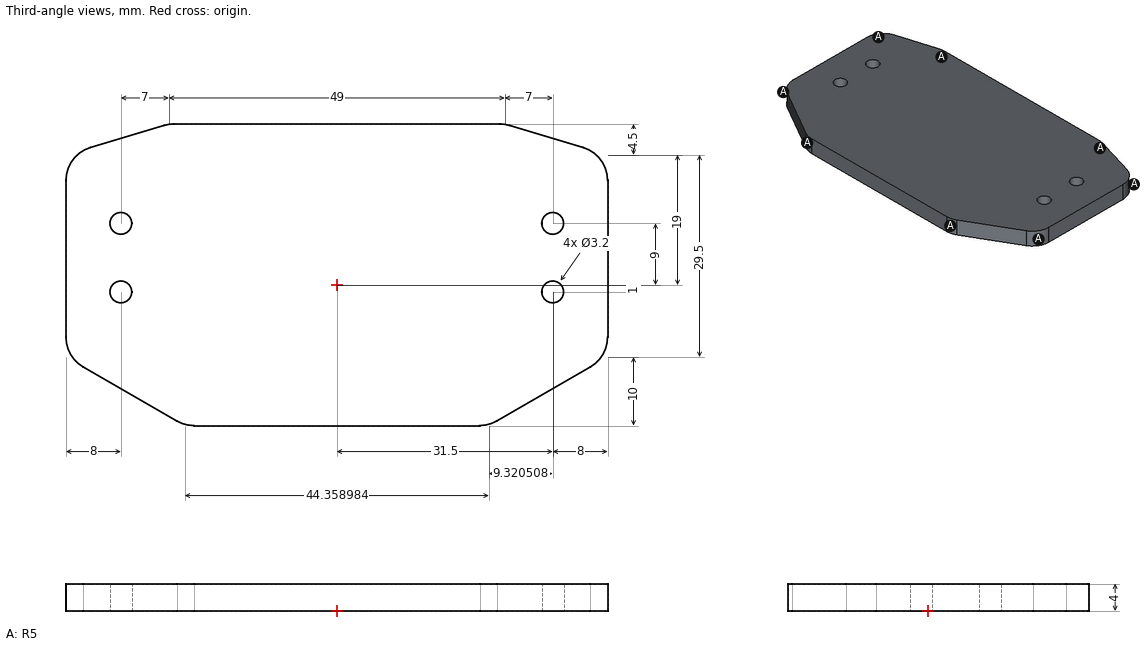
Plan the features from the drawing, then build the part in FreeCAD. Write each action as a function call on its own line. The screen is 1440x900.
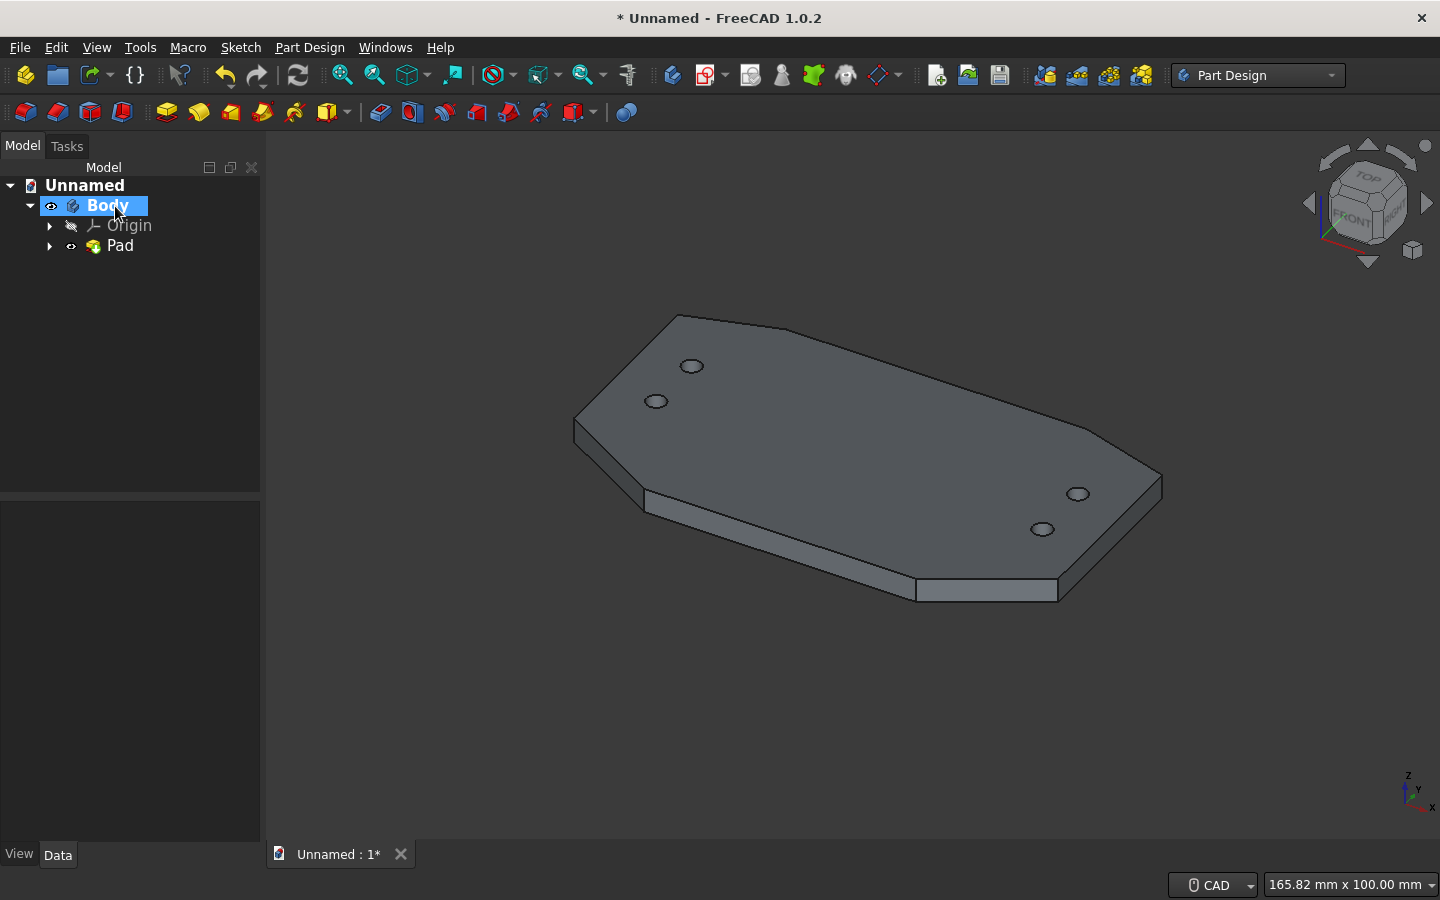
click(916, 590)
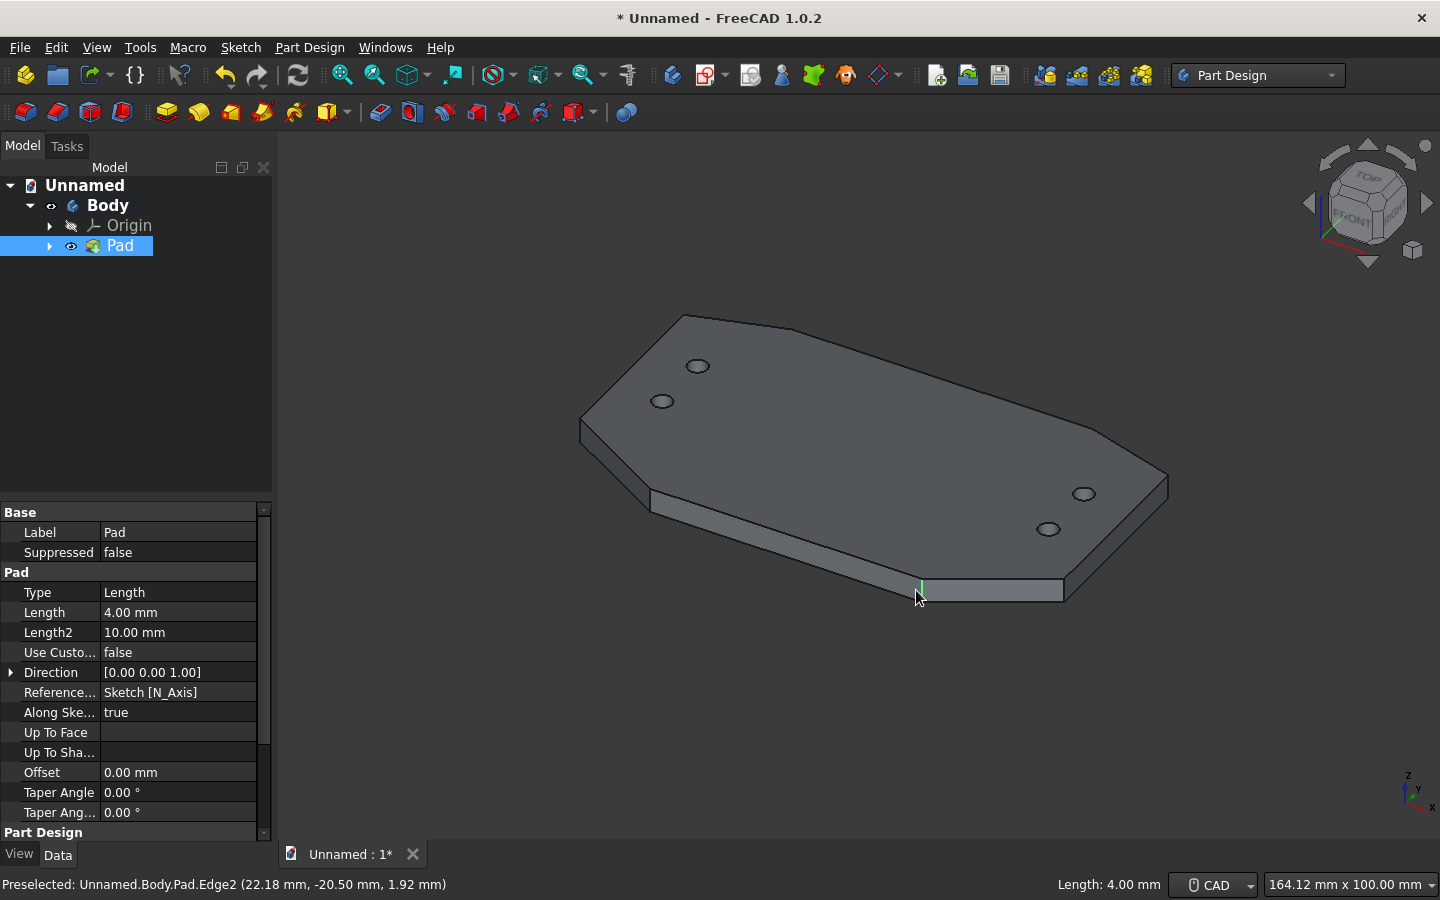
key(0)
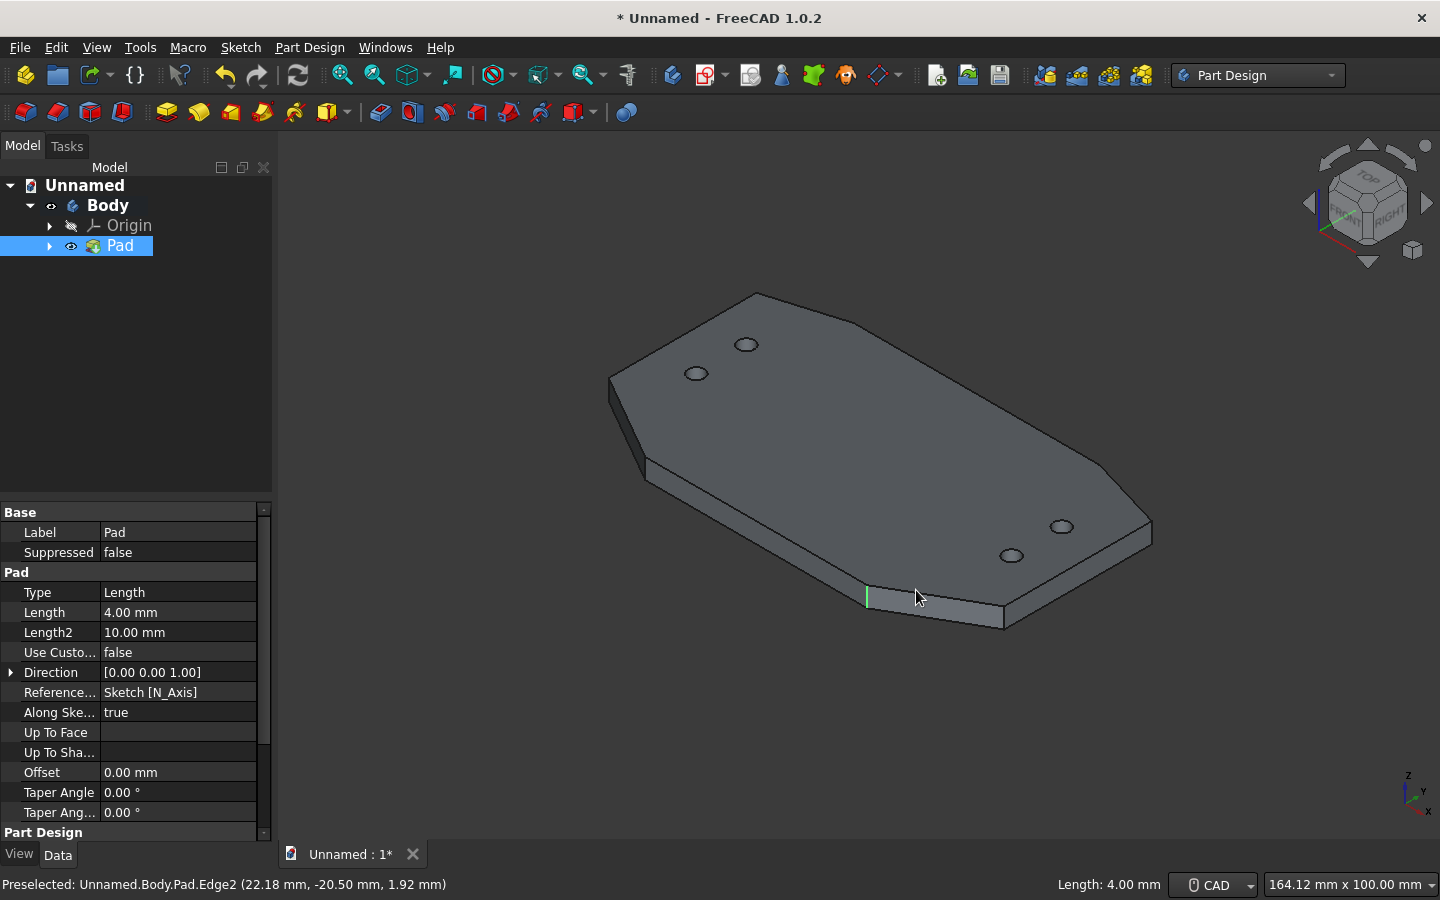
click(1004, 617, ctrl)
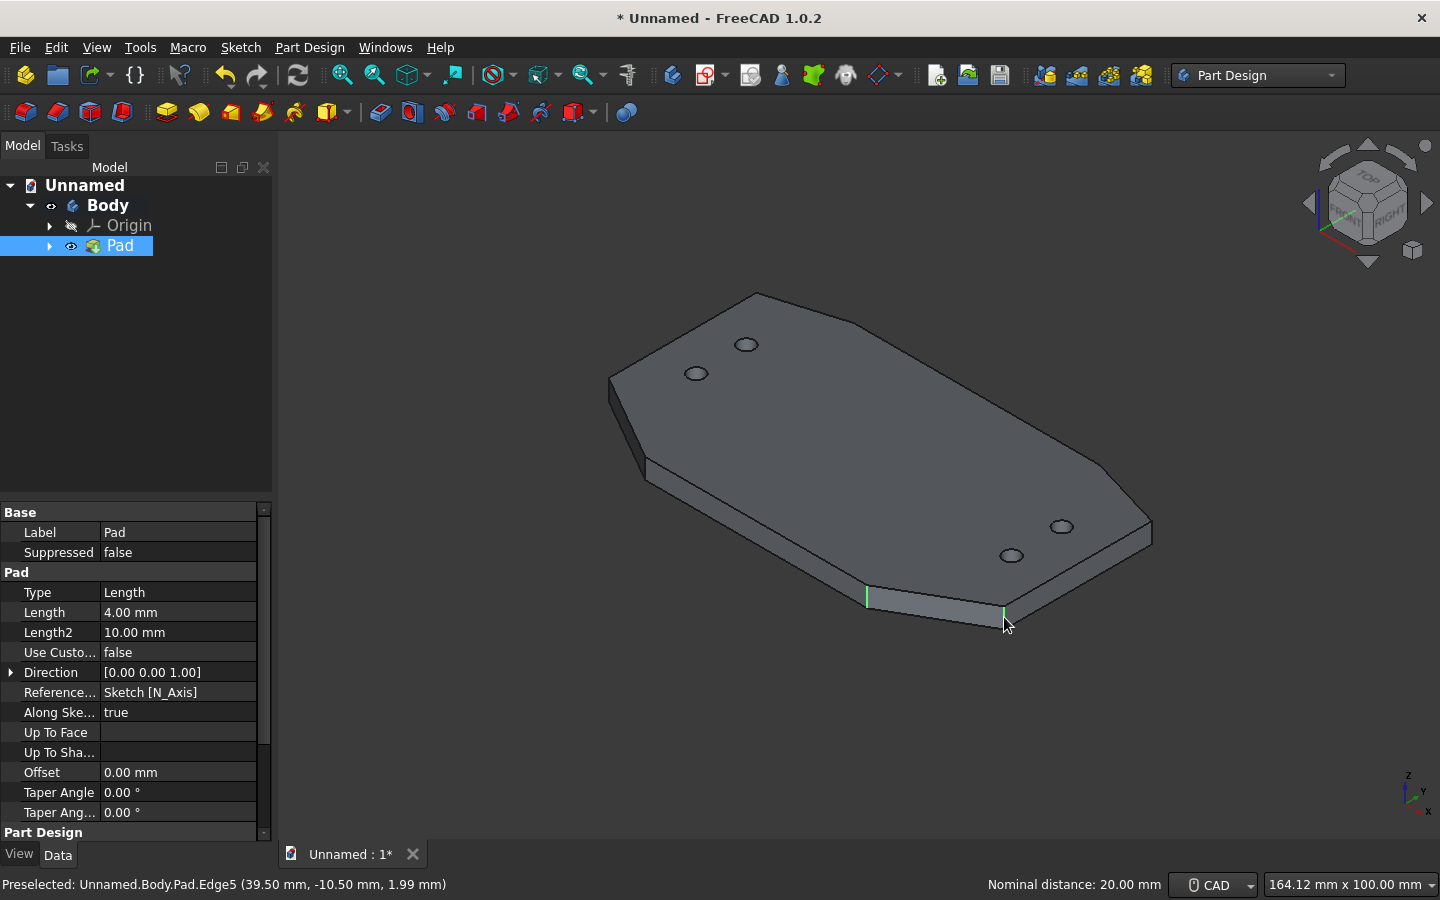
key(2)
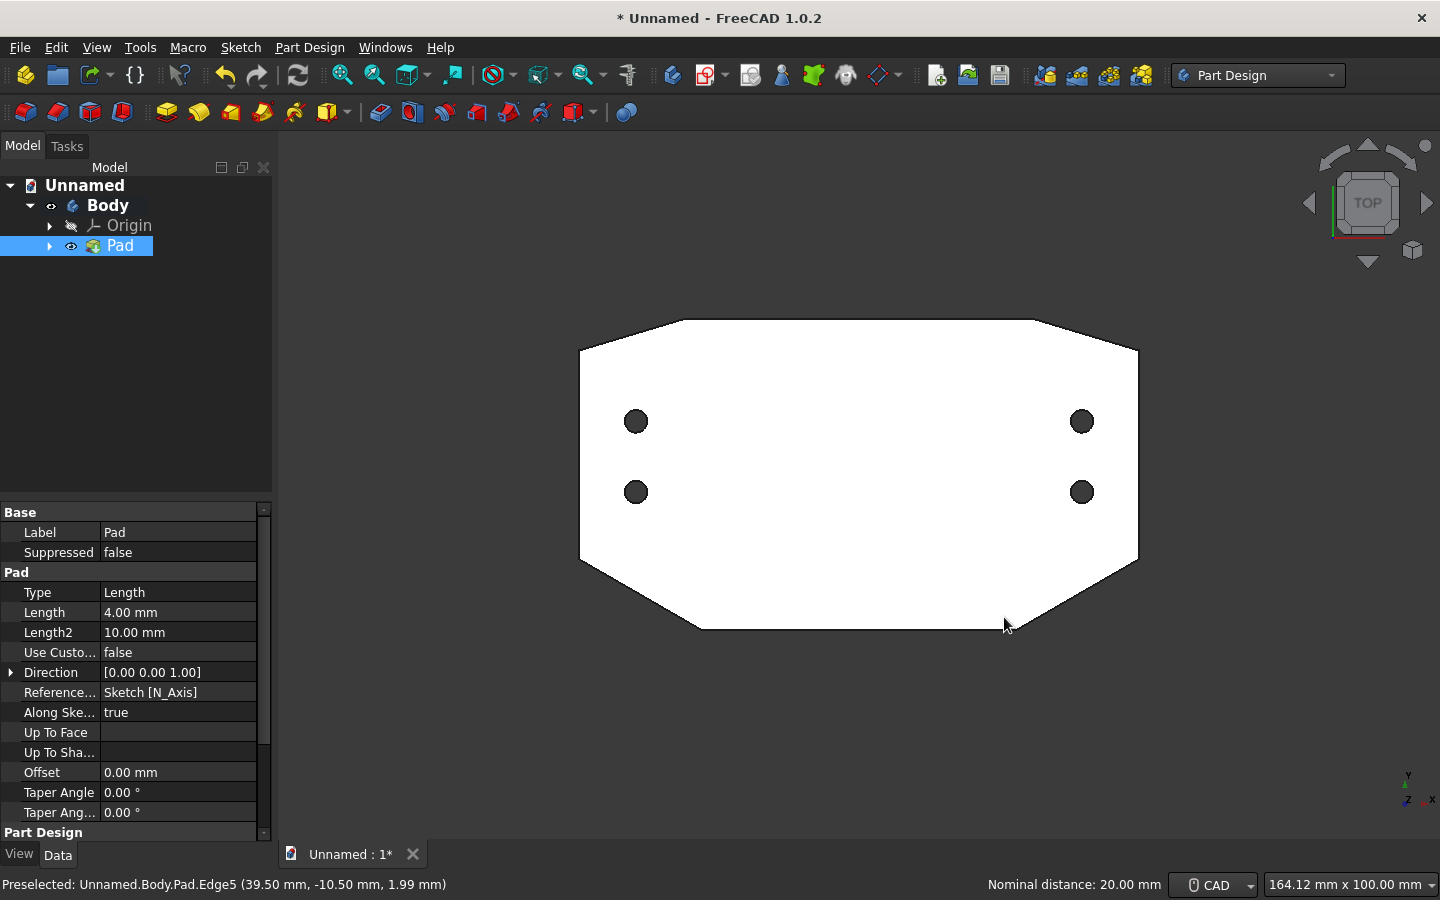
key(1)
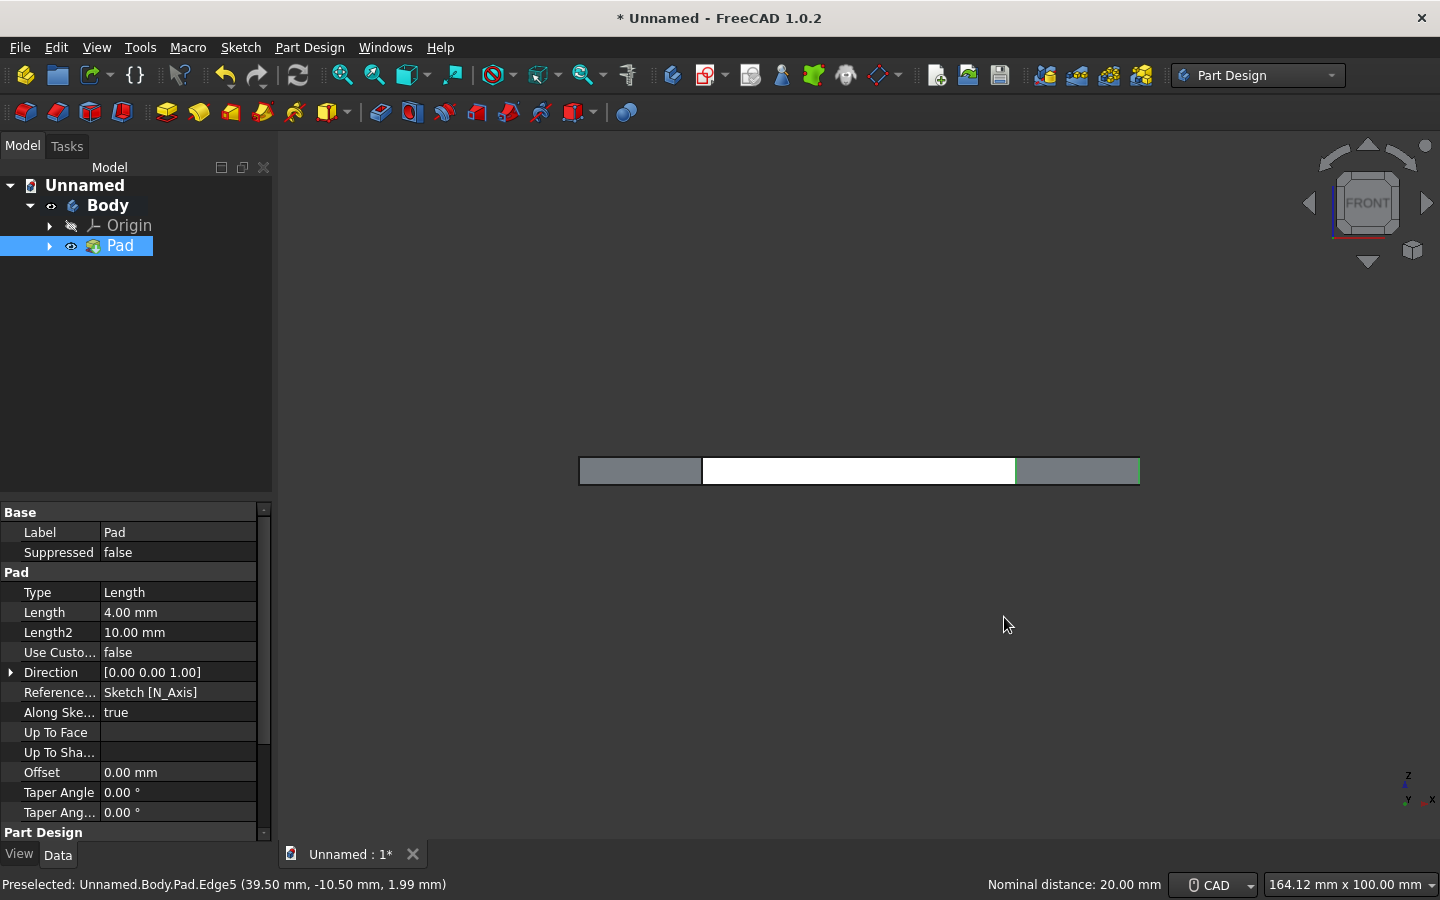
click(702, 470, ctrl)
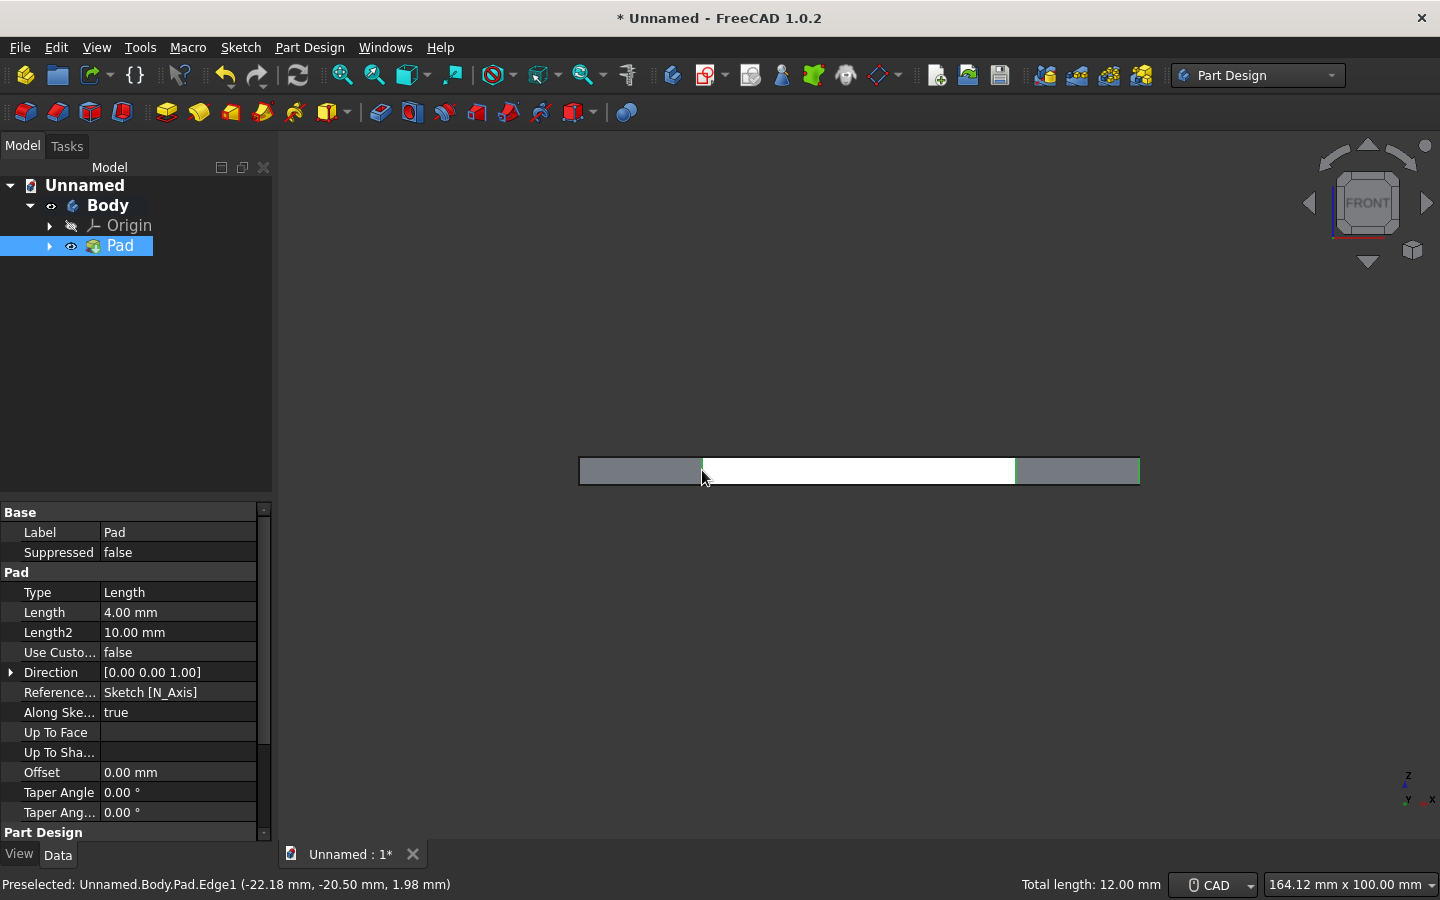
key(3)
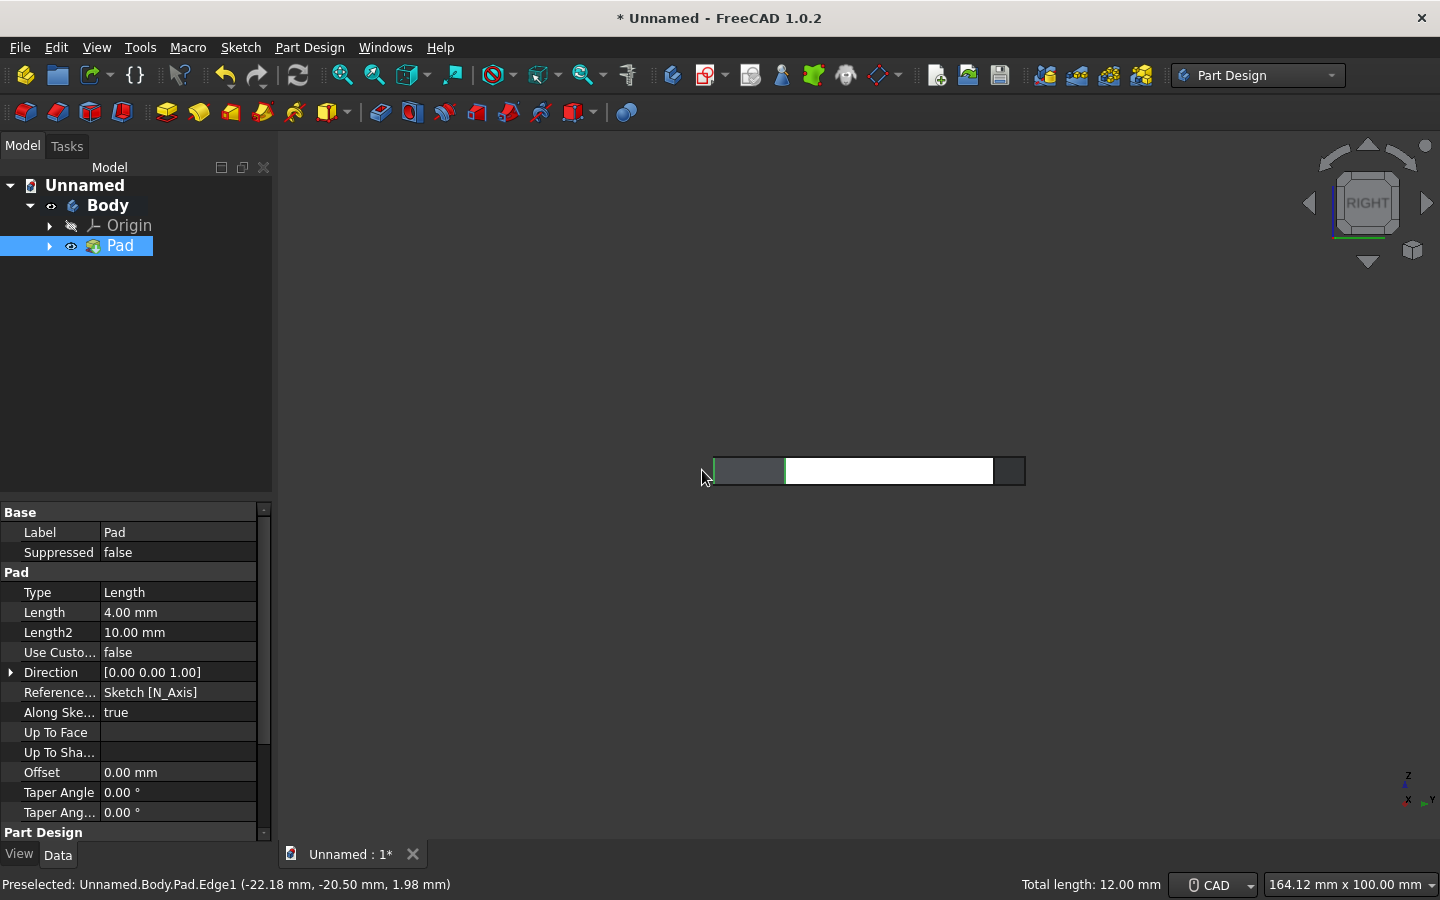
key(v)
key(f)